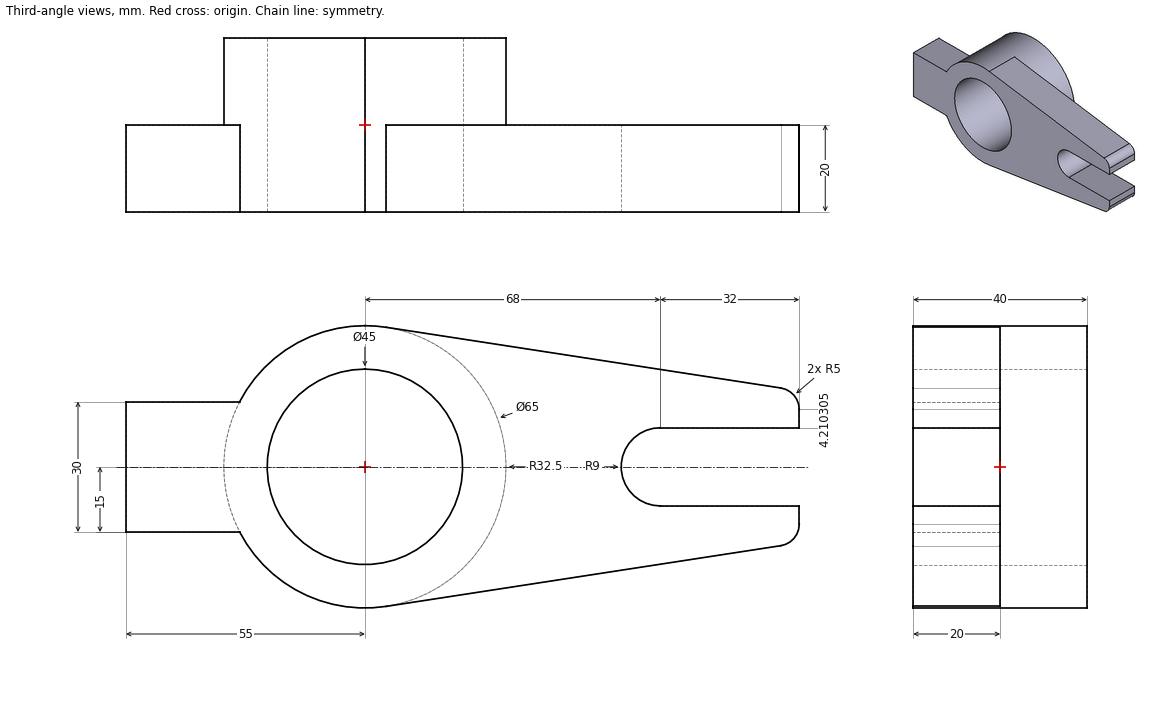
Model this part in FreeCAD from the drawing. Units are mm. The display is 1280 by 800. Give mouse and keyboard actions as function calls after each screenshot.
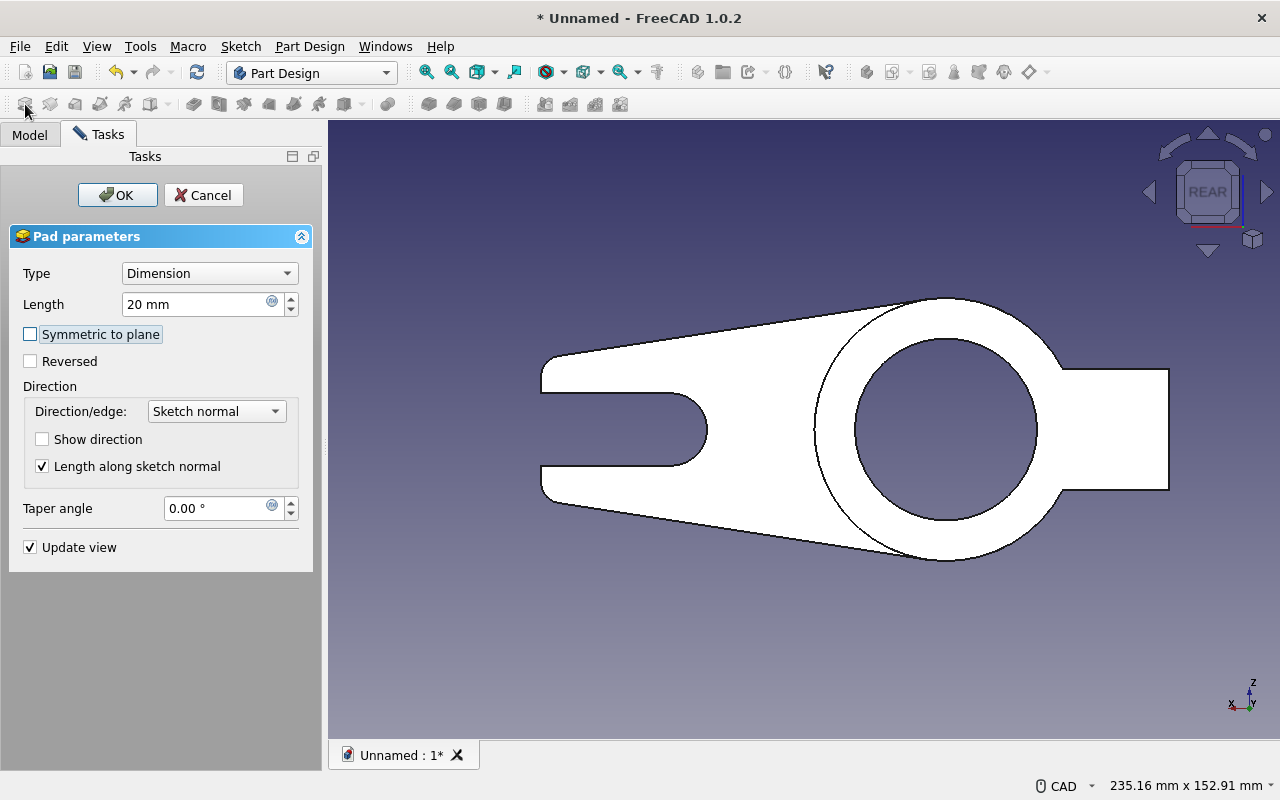
click(31, 361)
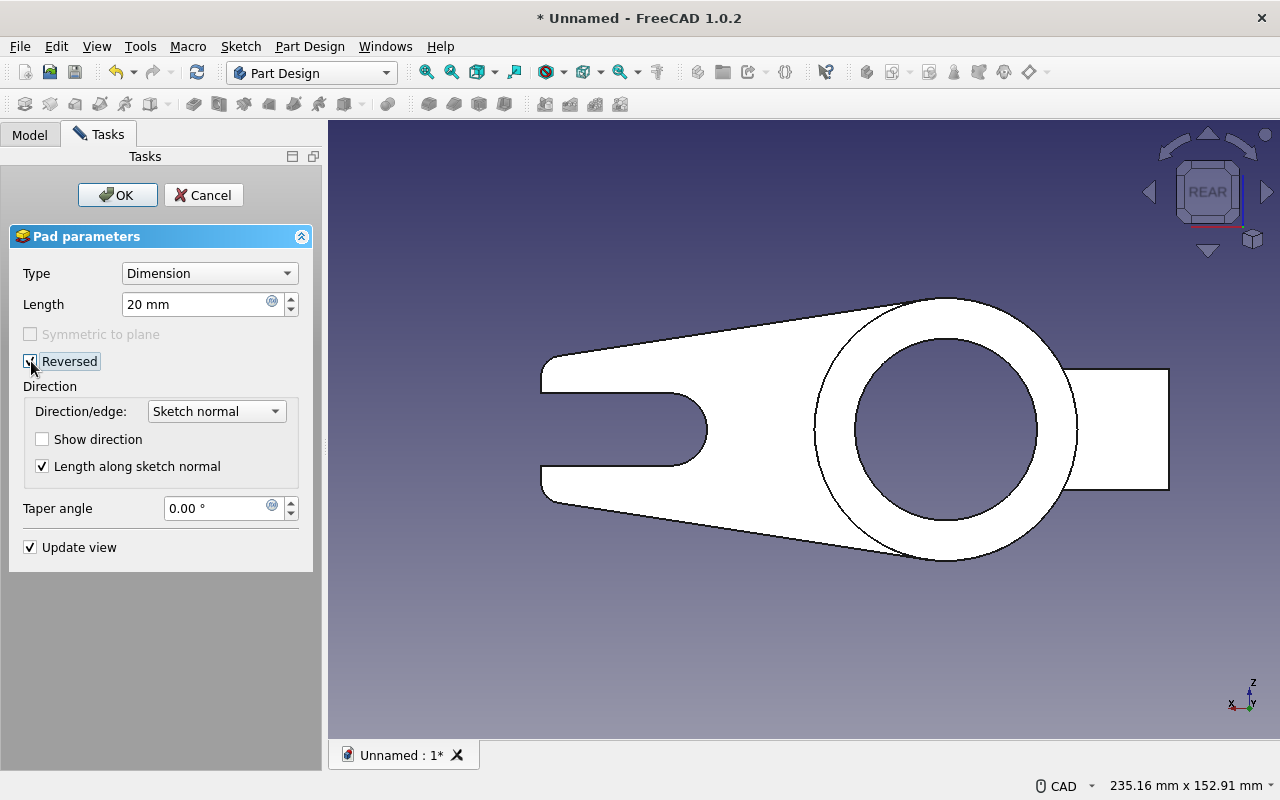
click(118, 195)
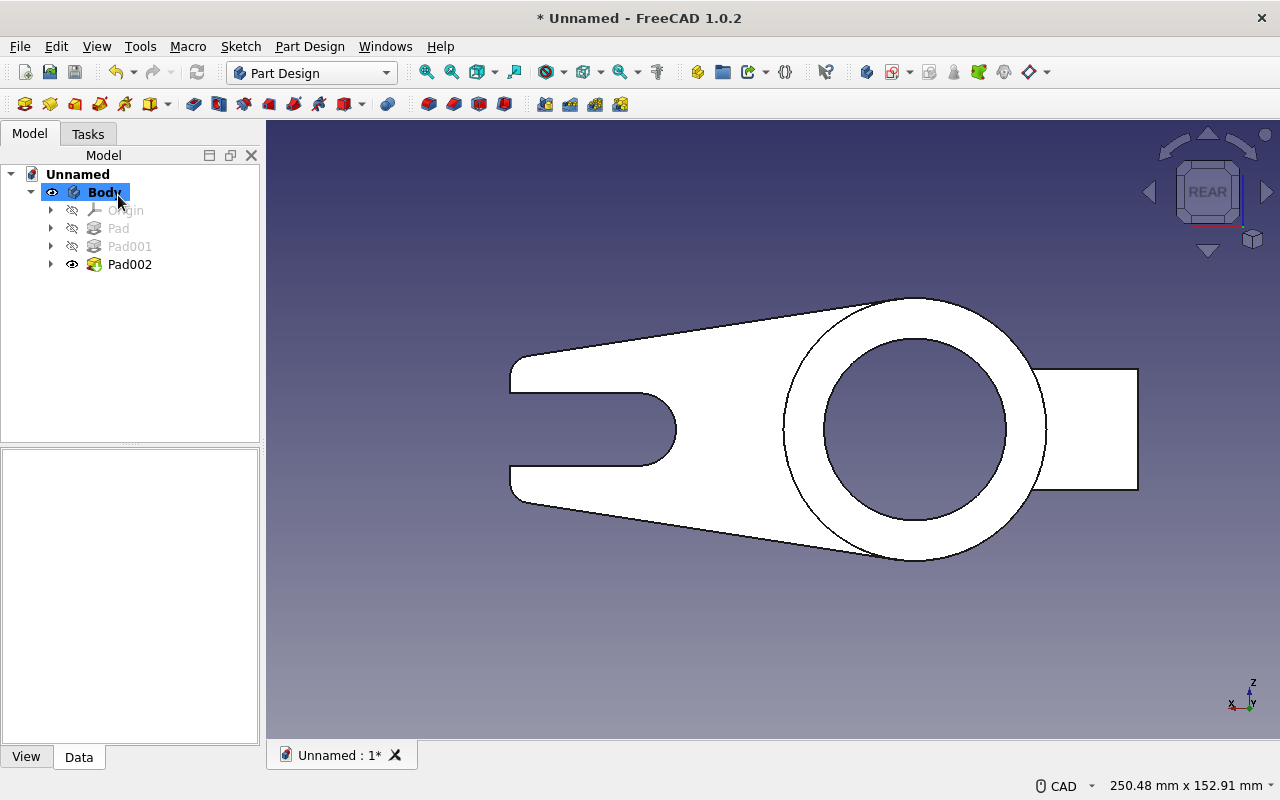
key(0)